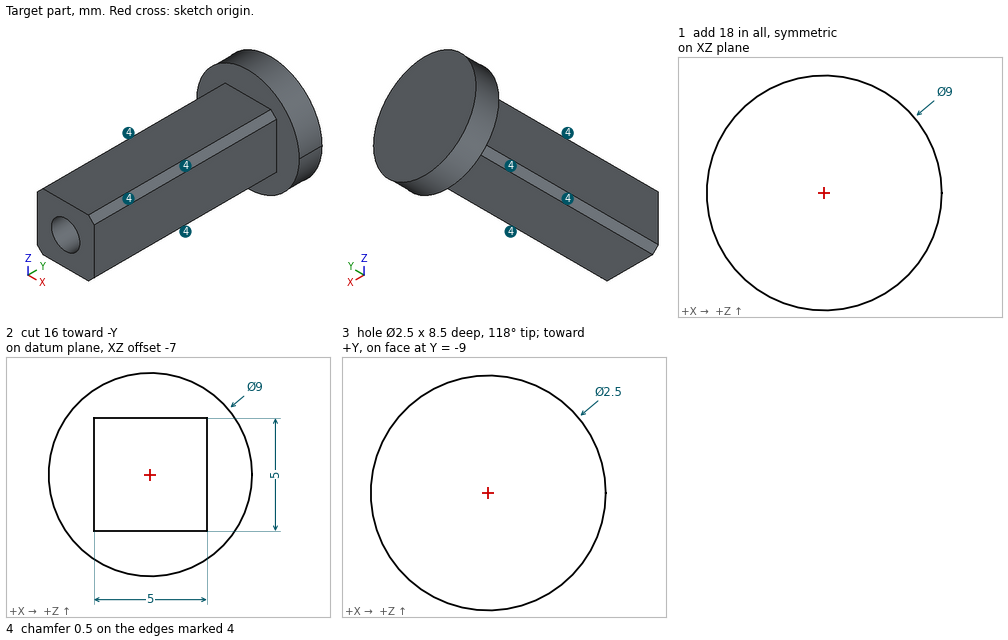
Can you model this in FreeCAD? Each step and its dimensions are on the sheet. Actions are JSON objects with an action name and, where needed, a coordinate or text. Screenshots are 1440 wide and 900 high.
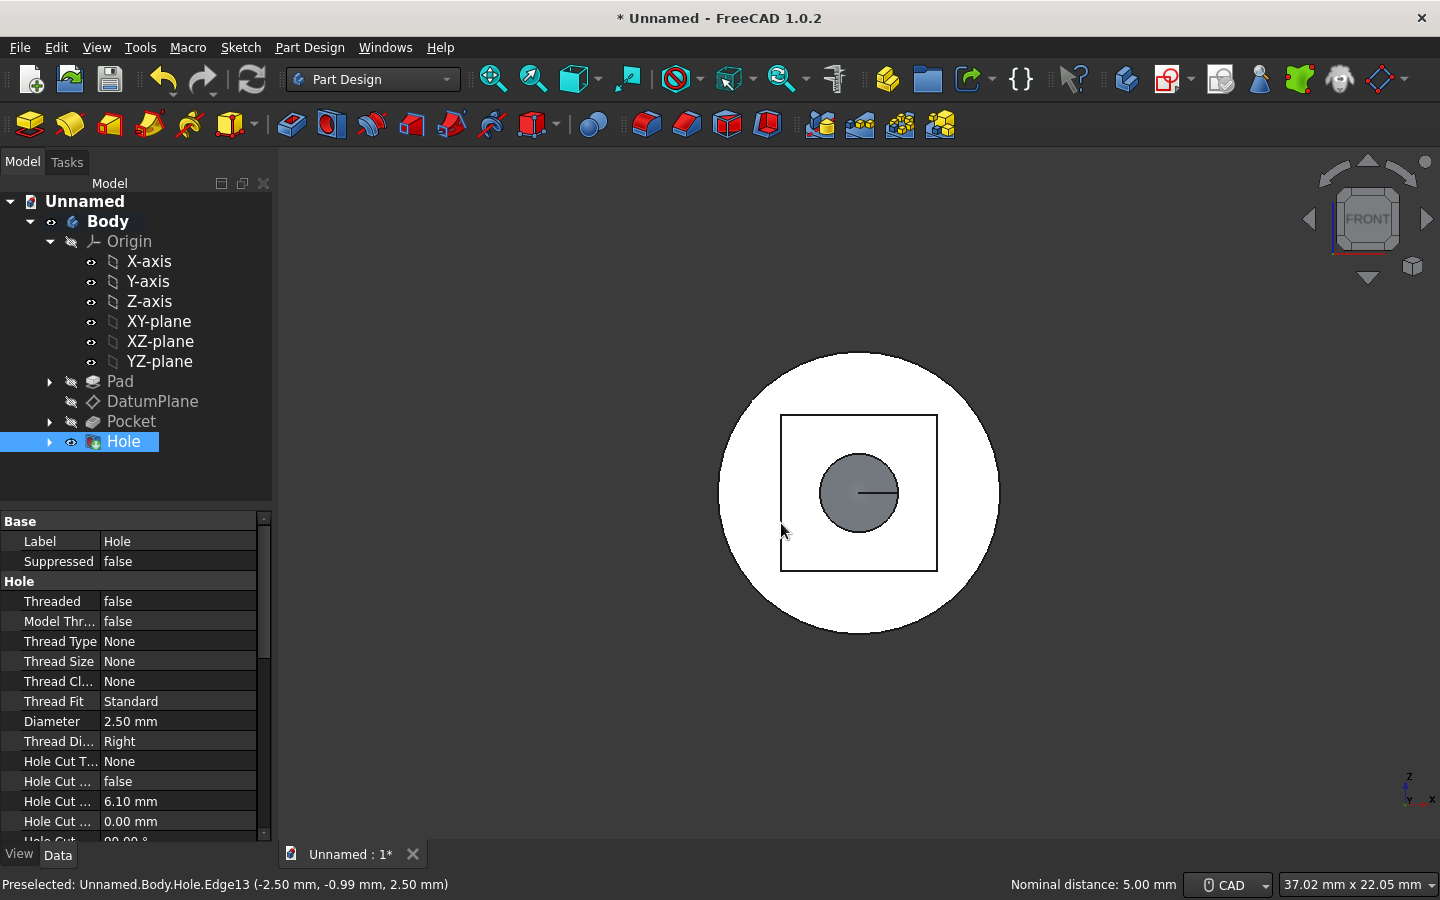
{"action": "left_click", "coordinate": [494, 80]}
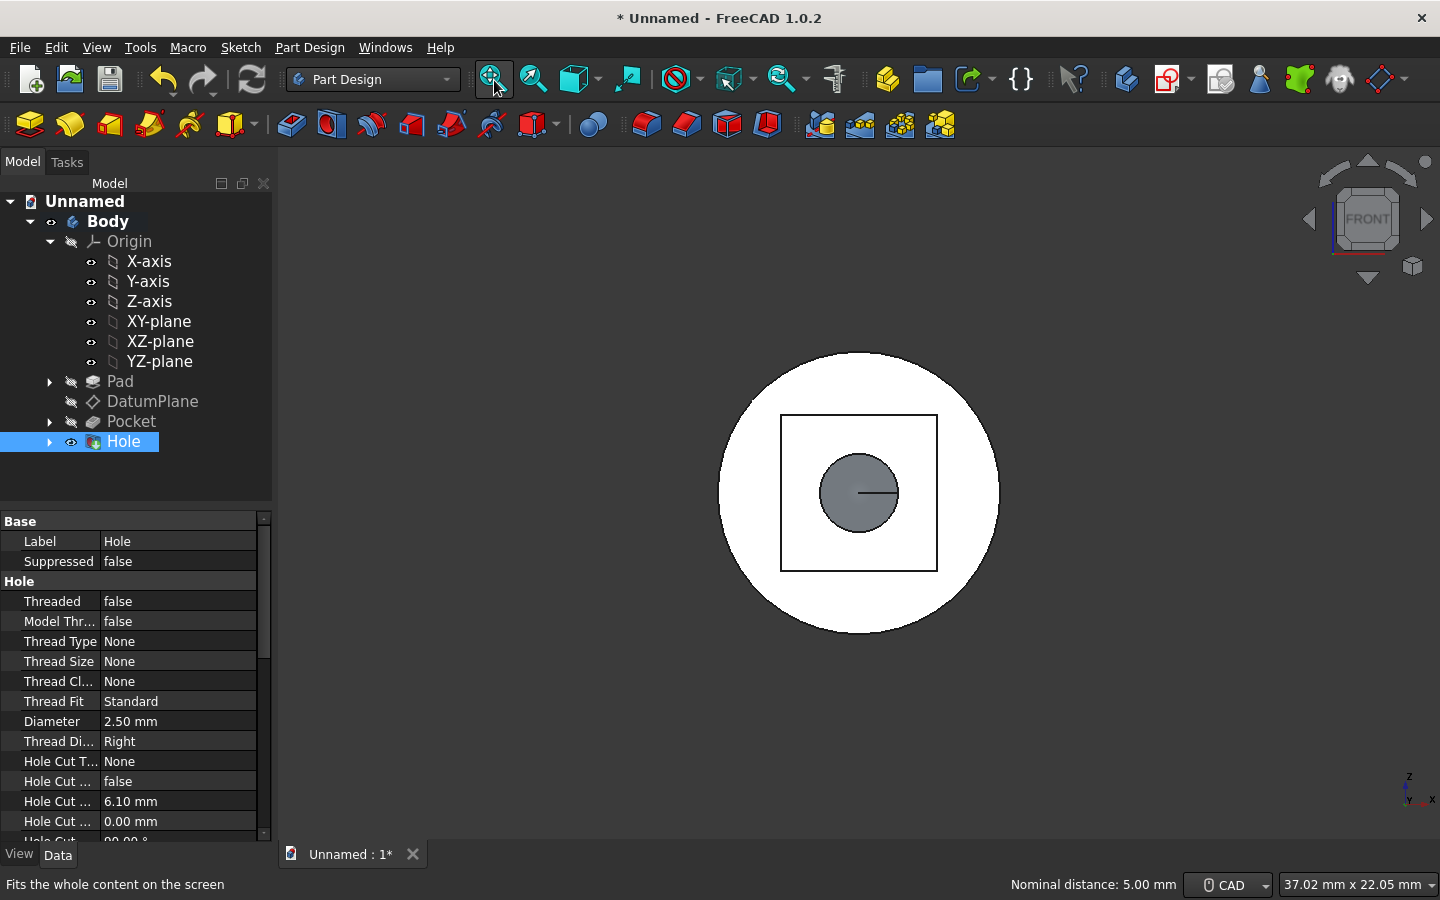
{"action": "key", "text": "3"}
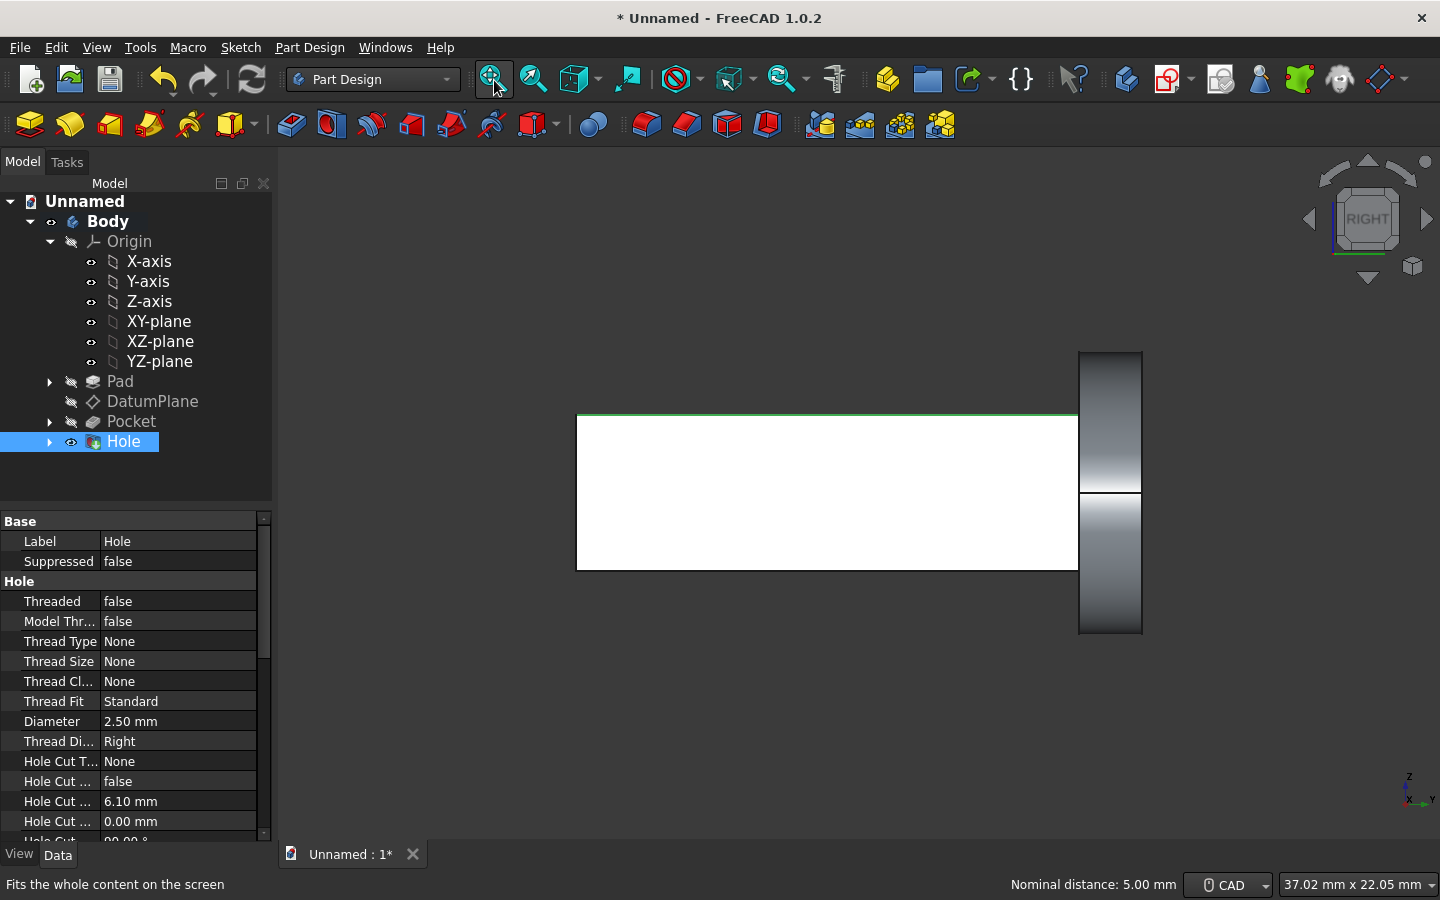
{"action": "left_click", "coordinate": [828, 570], "text": "ctrl"}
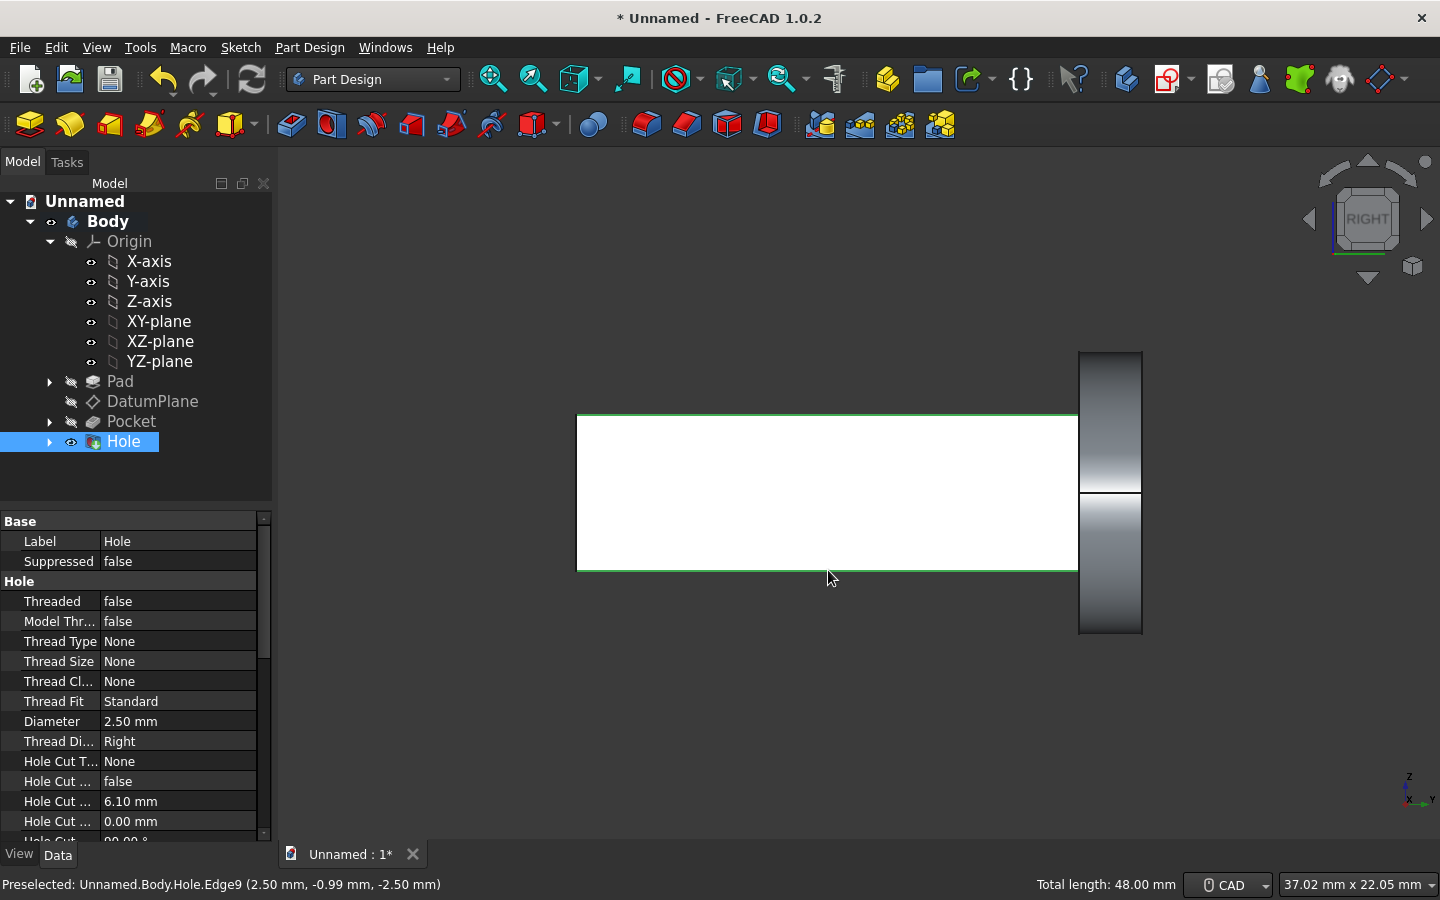
{"action": "key", "text": "5"}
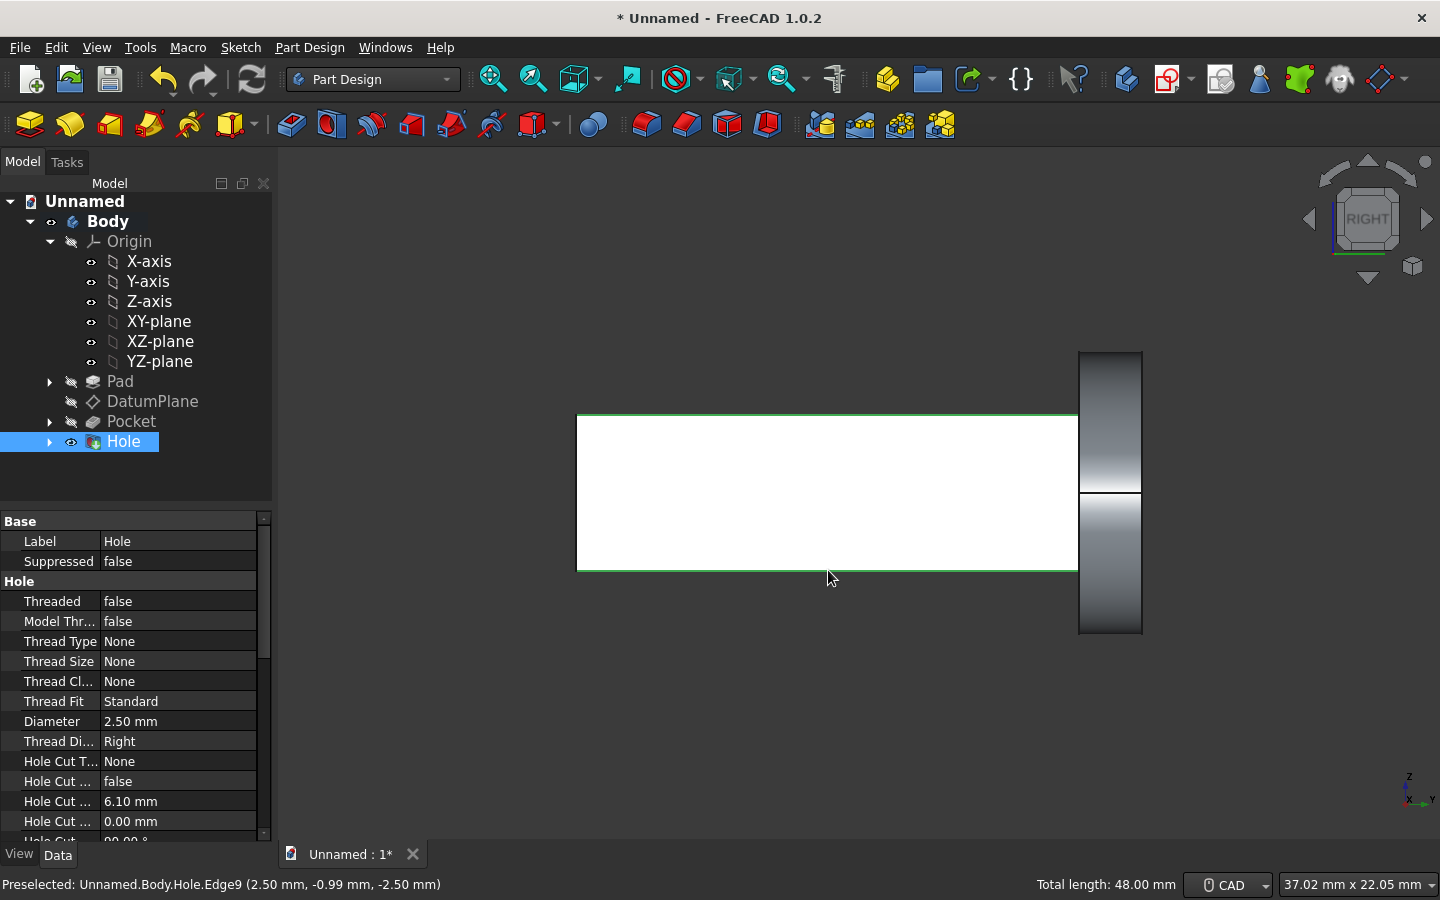
{"action": "left_click", "coordinate": [781, 461], "text": "ctrl"}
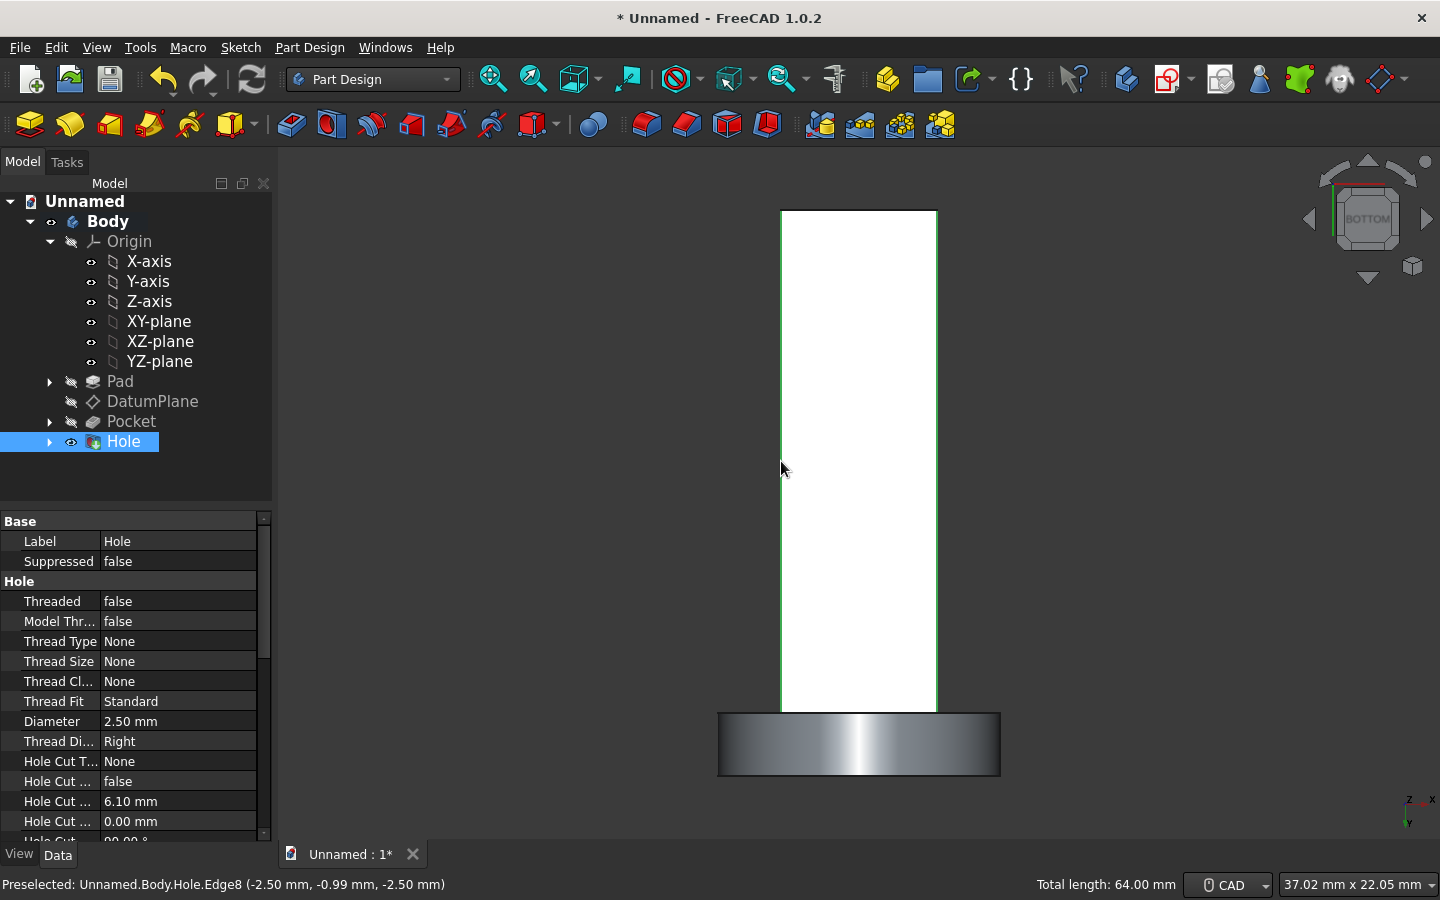
{"action": "left_click", "coordinate": [688, 124]}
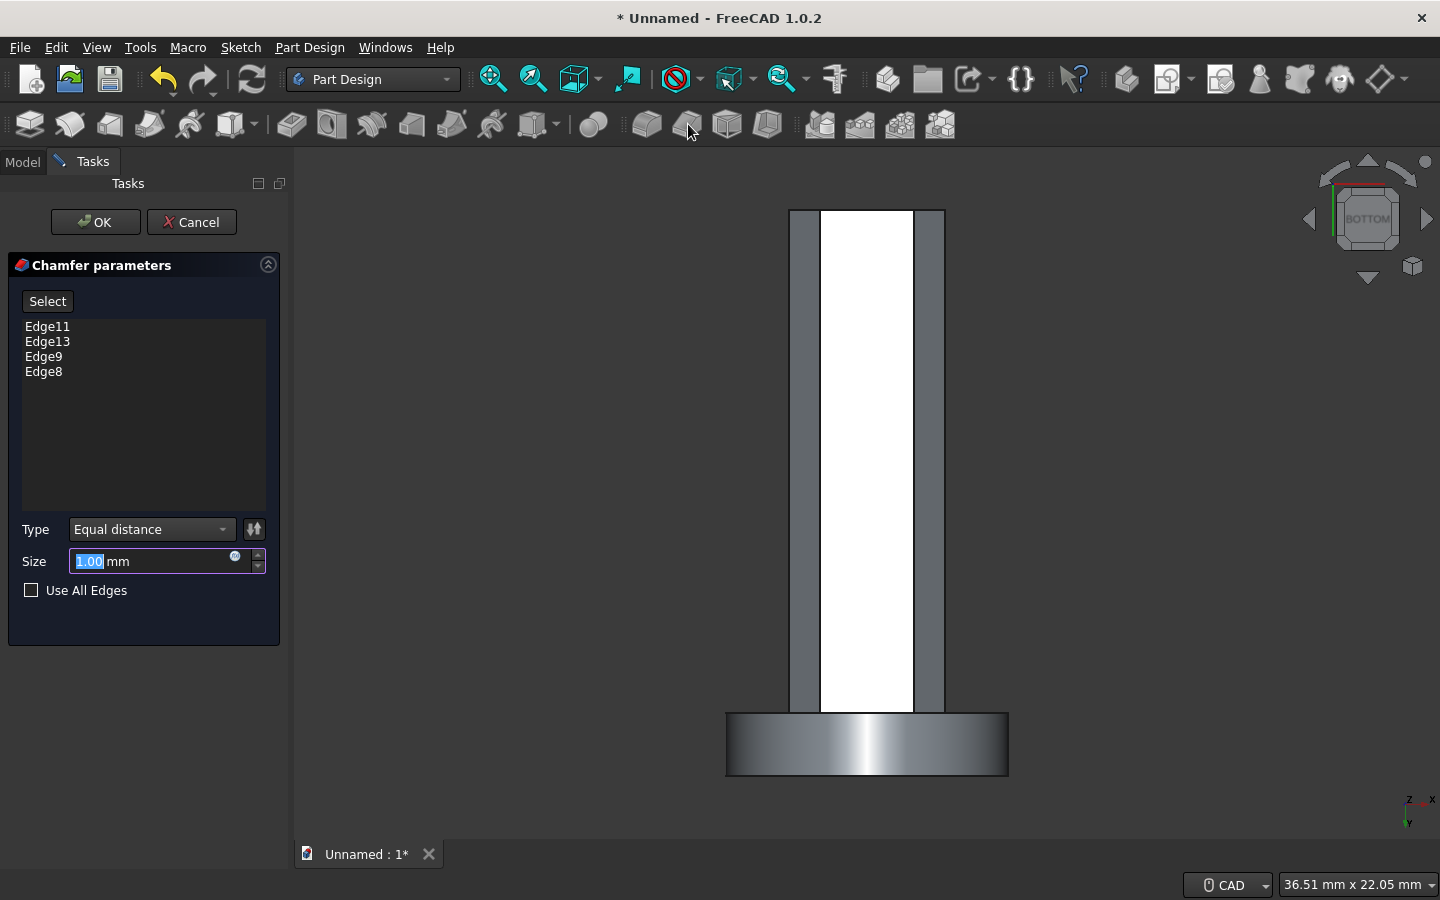
{"action": "type", "text": "0.5"}
{"action": "key", "text": "Tab"}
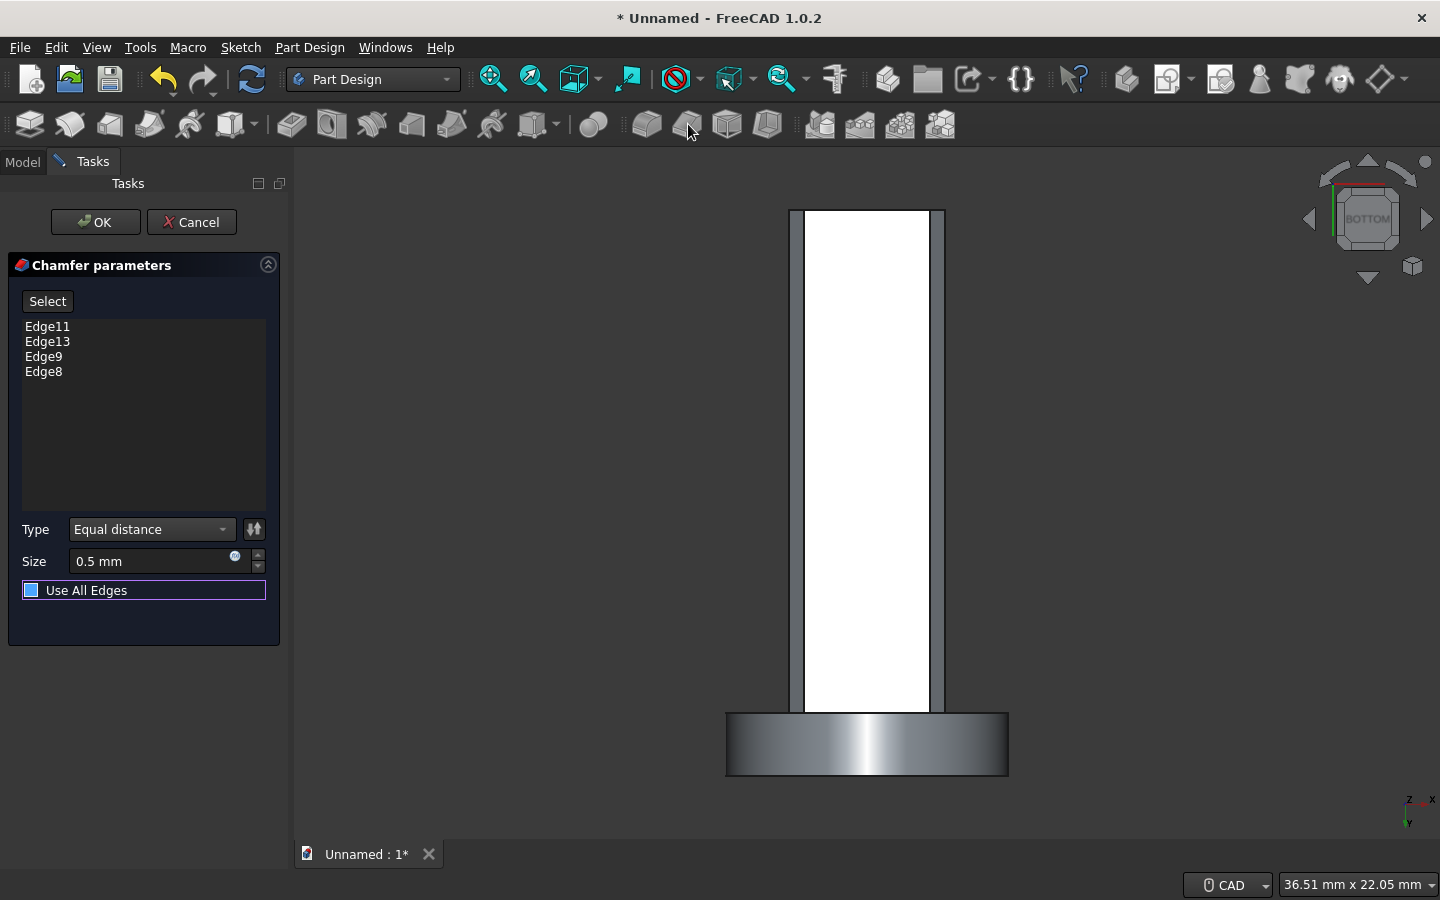
{"action": "left_click", "coordinate": [96, 222]}